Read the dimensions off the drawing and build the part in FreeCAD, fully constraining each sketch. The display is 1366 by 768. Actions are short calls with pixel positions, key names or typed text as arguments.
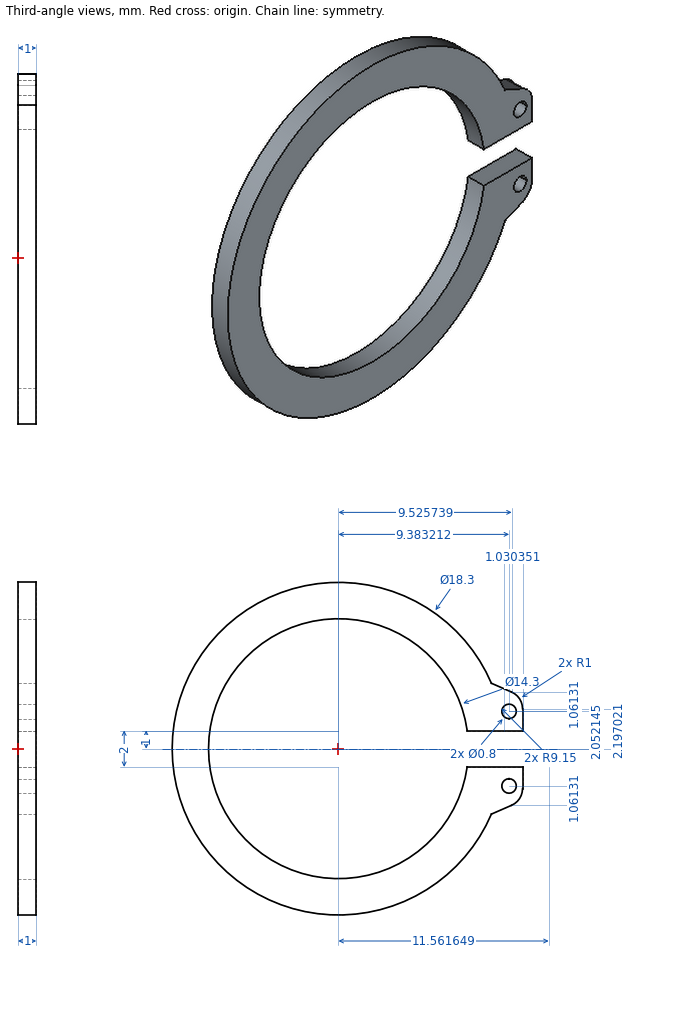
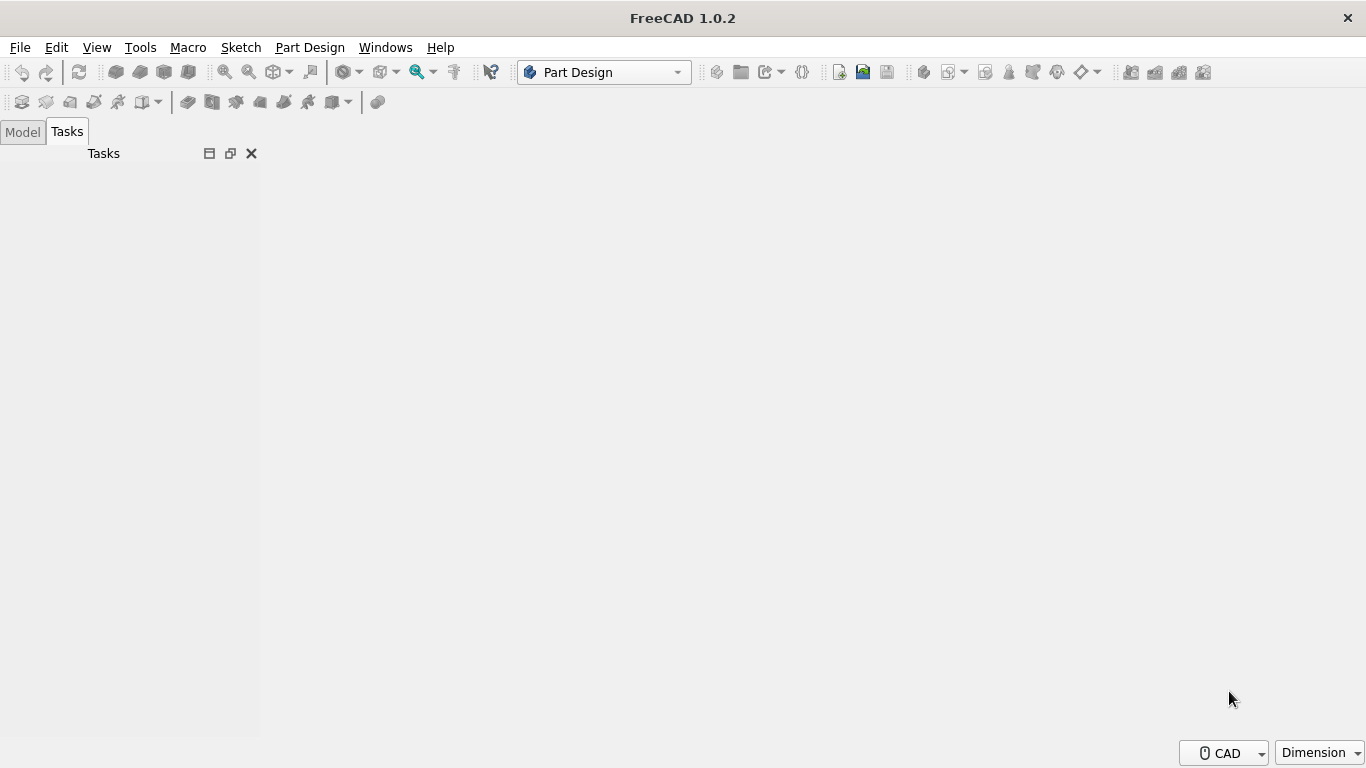
click(840, 72)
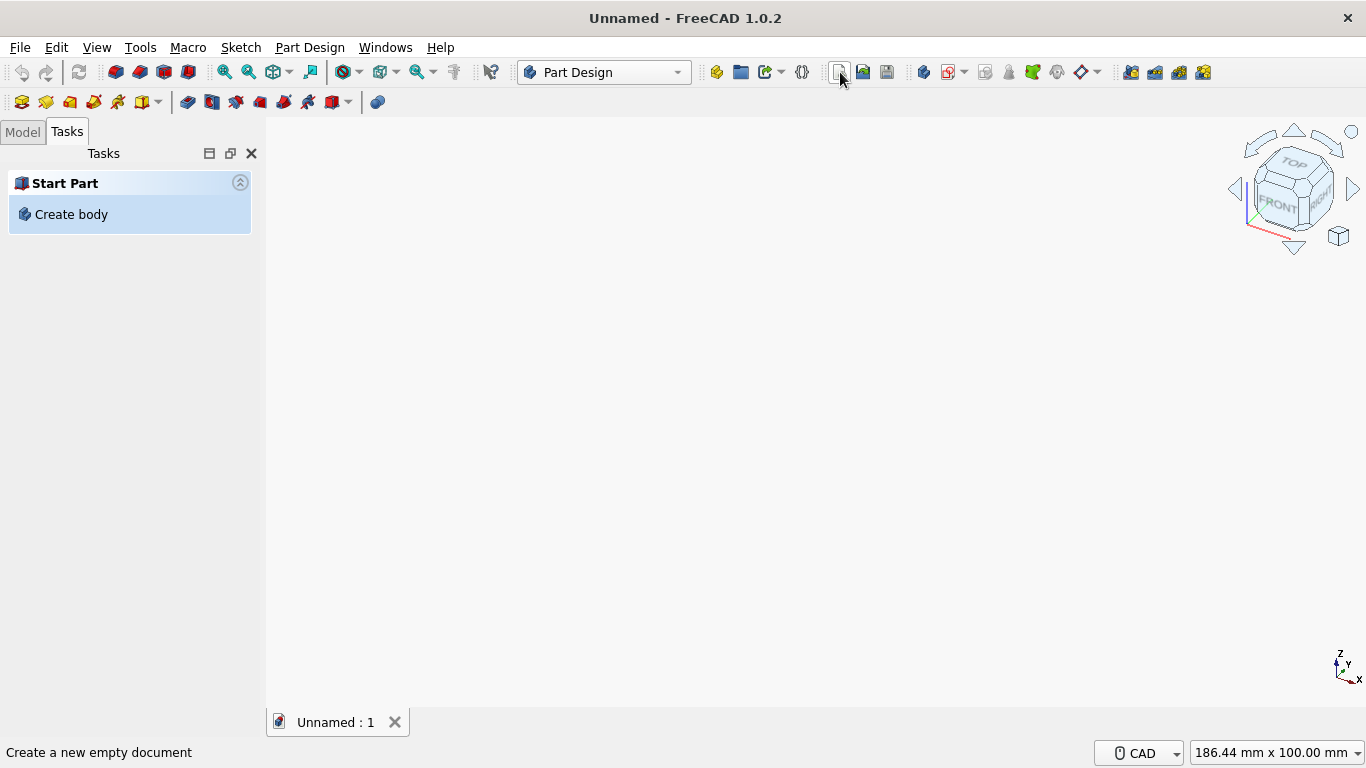
click(948, 72)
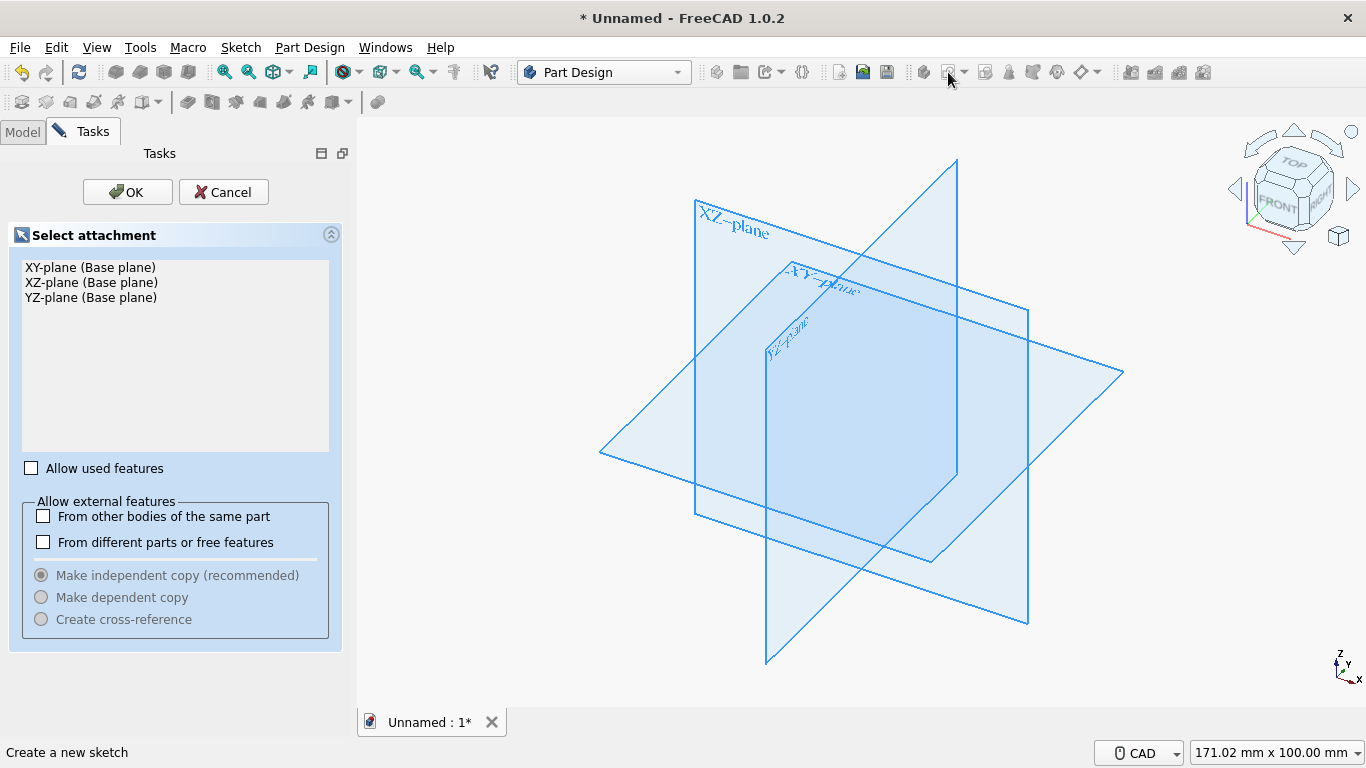
click(82, 298)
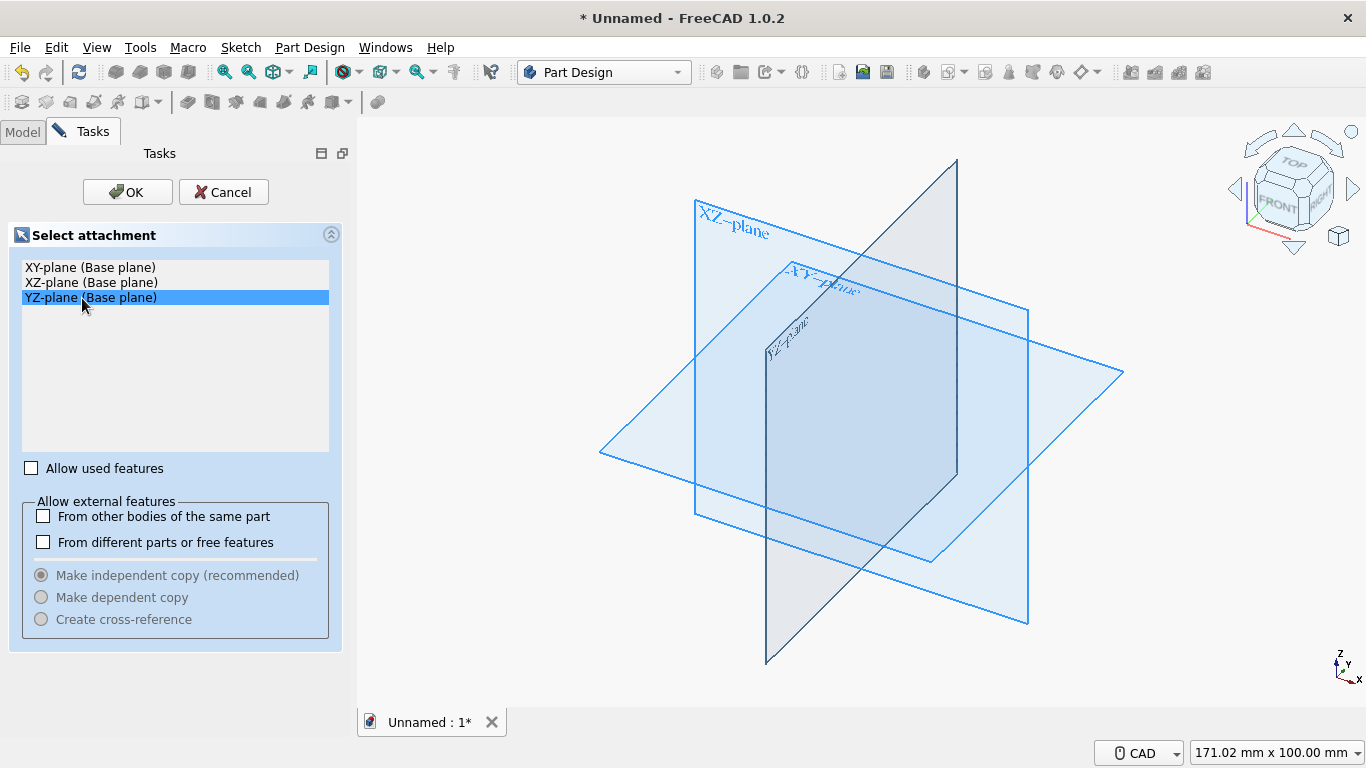
click(128, 192)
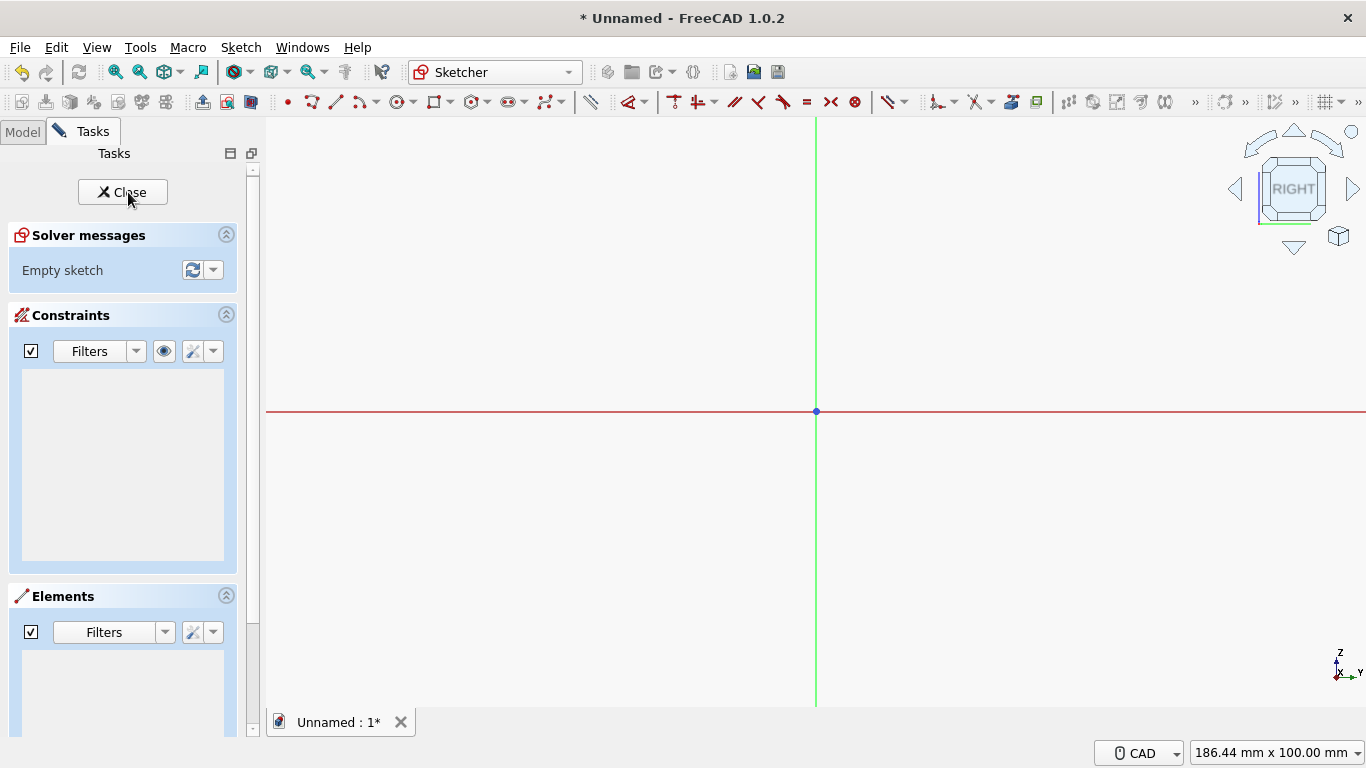
scroll(846, 412, up, 6)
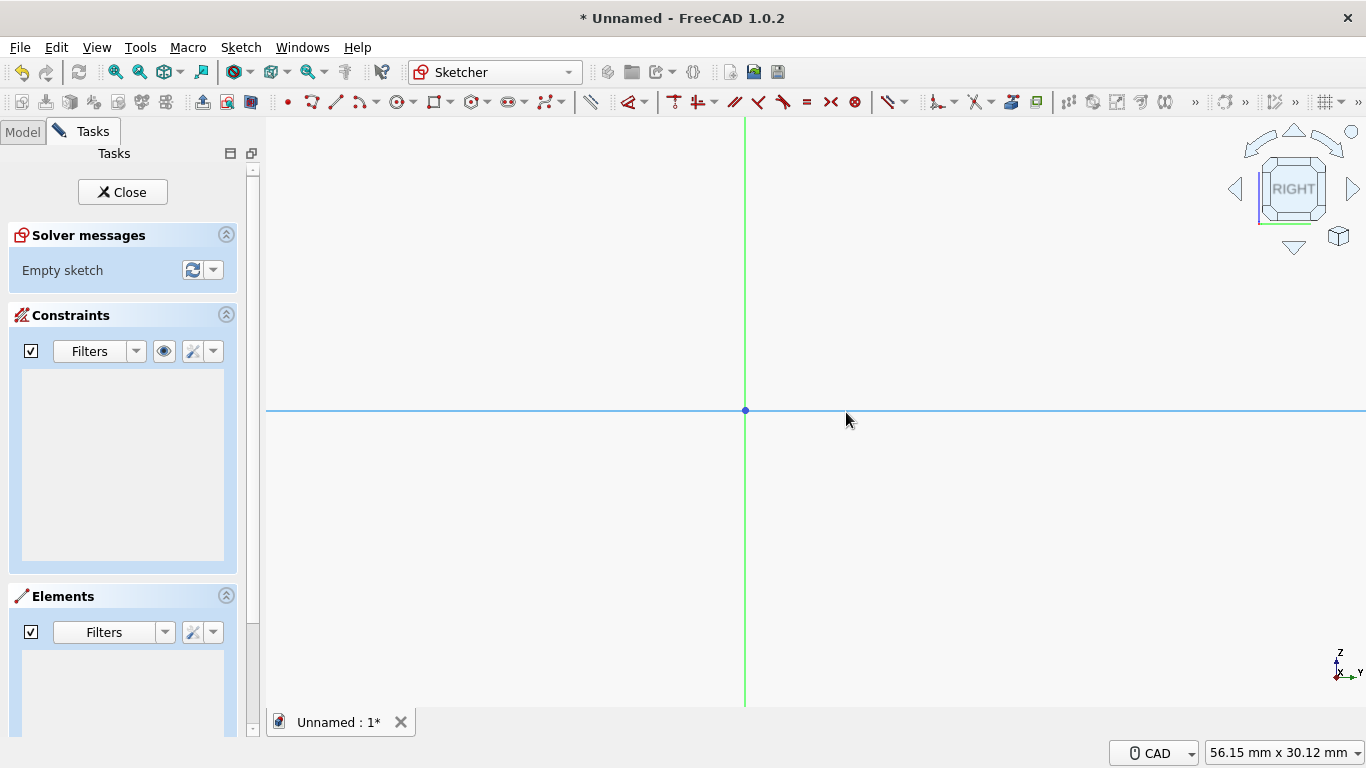
click(398, 102)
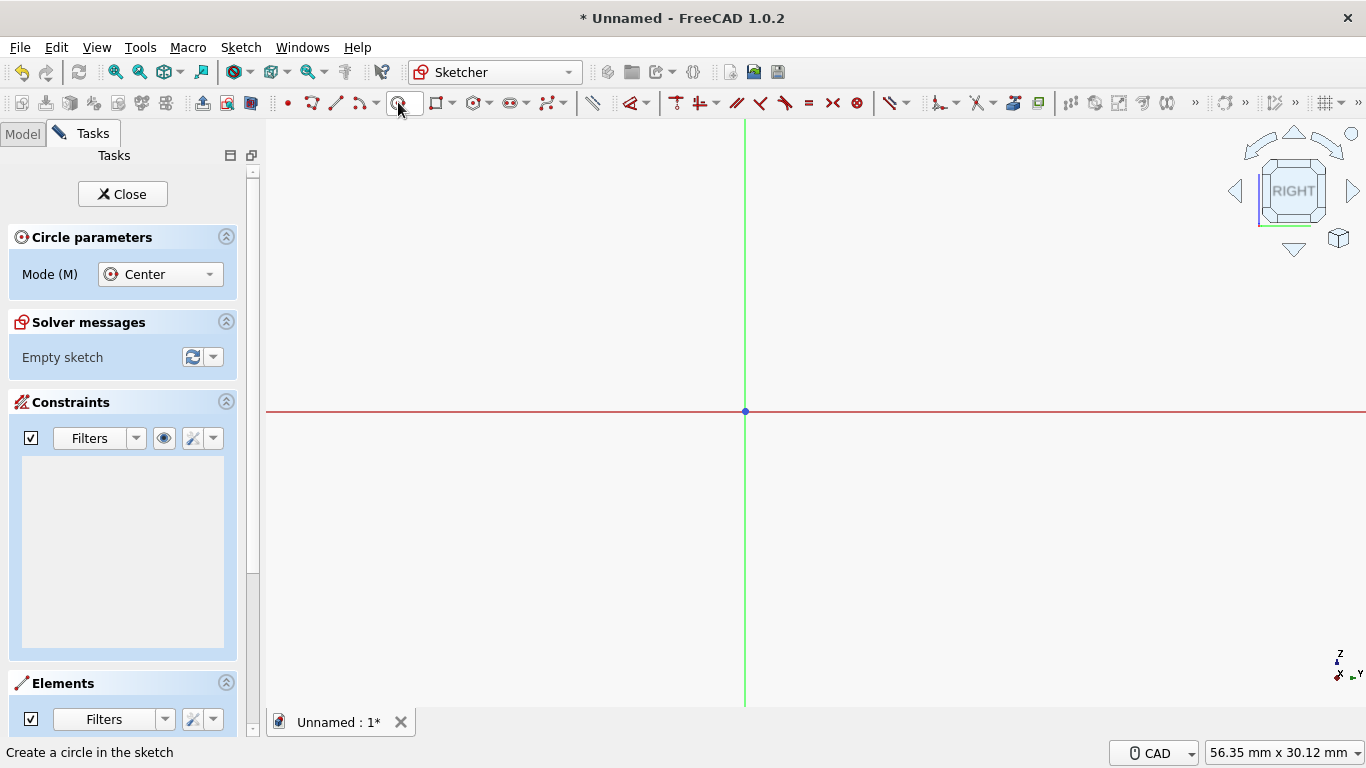
click(745, 412)
click(872, 286)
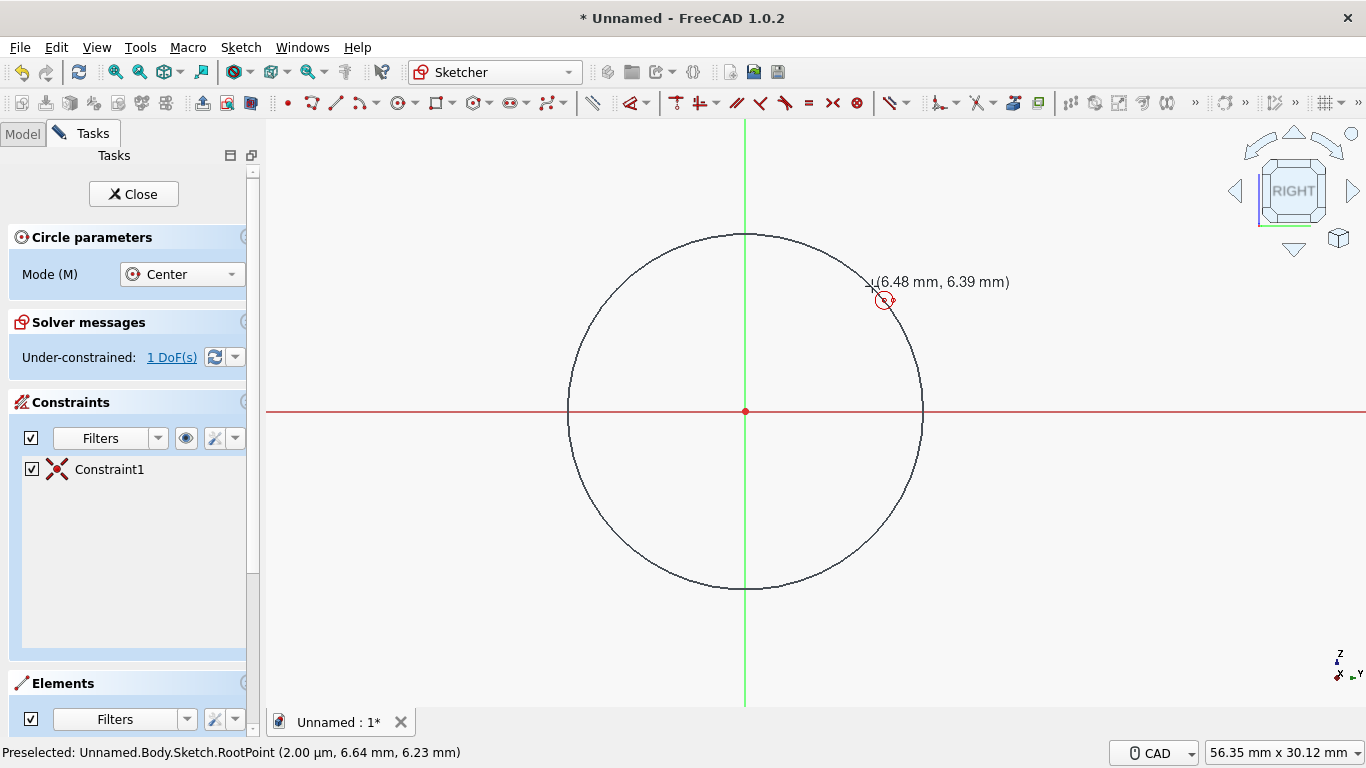
click(745, 412)
click(844, 313)
key(Escape)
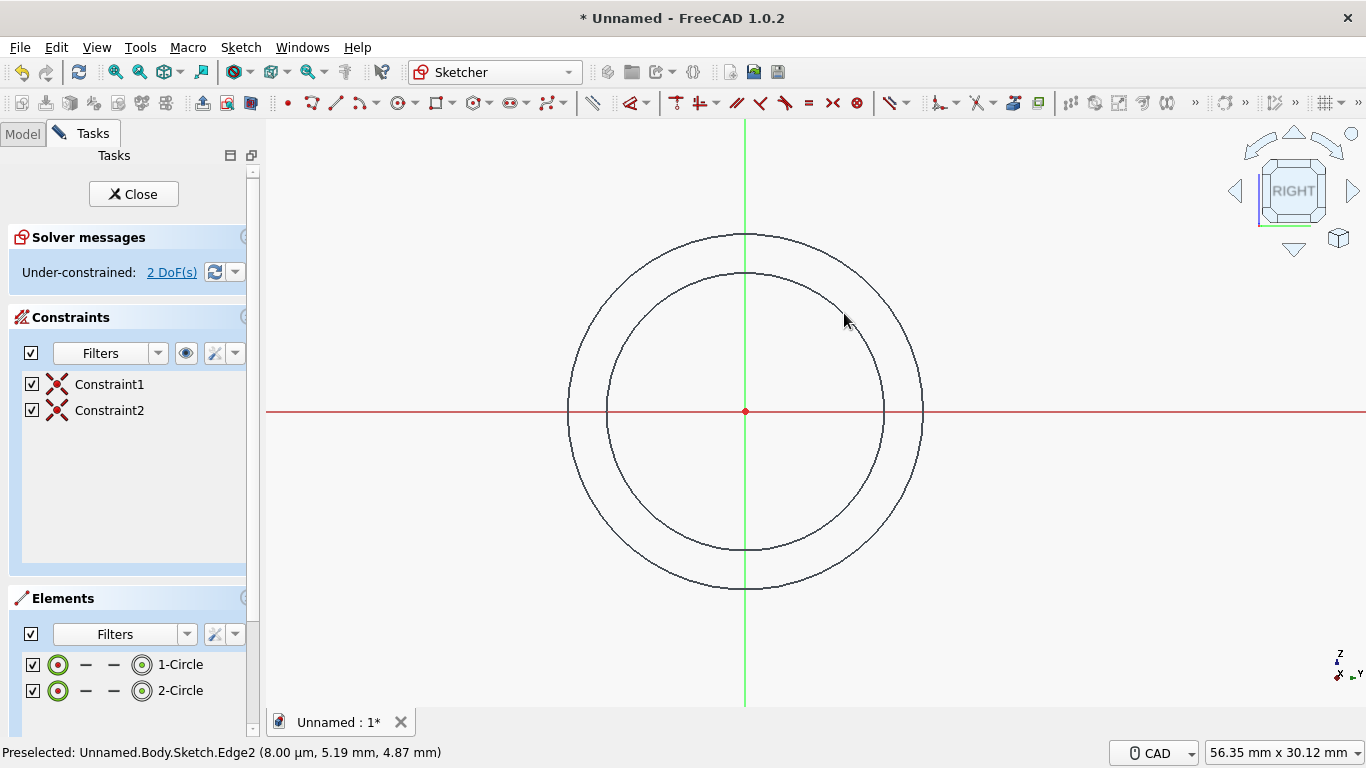
click(871, 286)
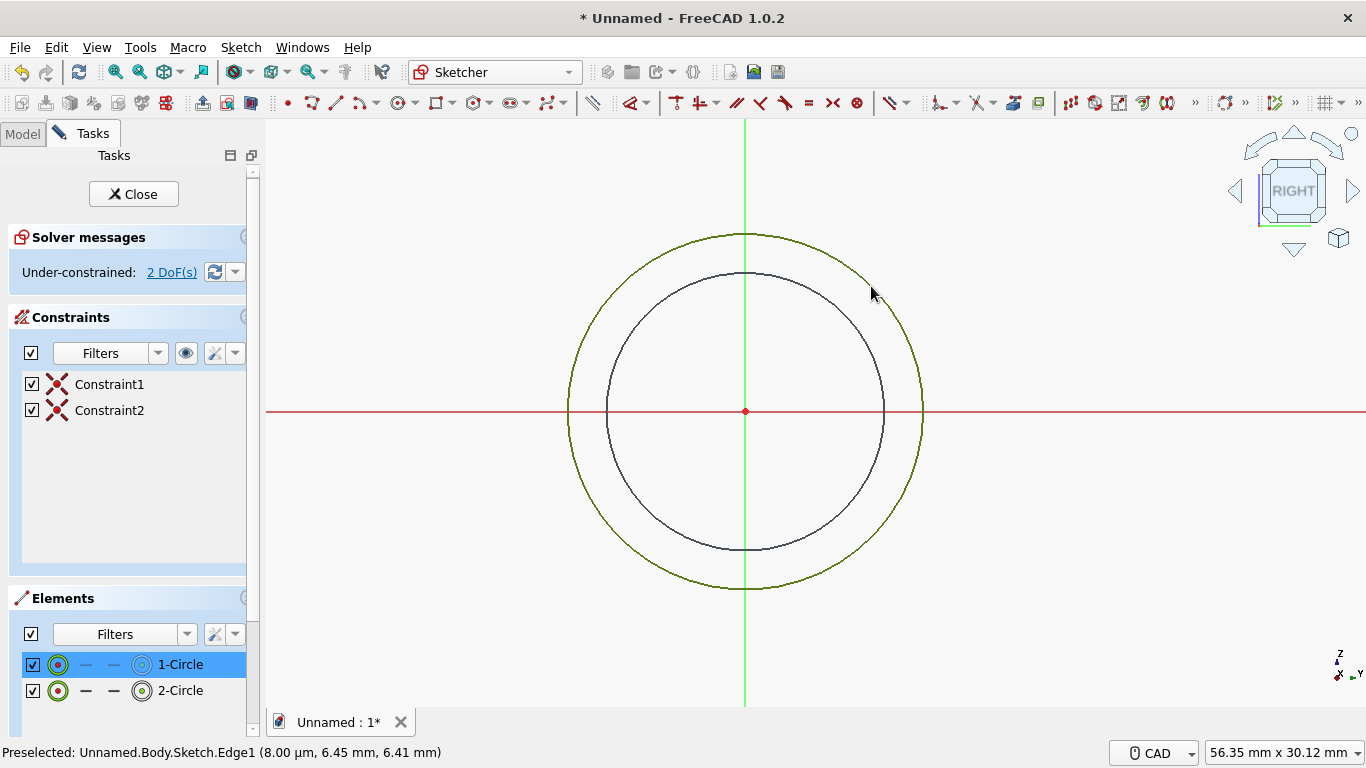
click(648, 104)